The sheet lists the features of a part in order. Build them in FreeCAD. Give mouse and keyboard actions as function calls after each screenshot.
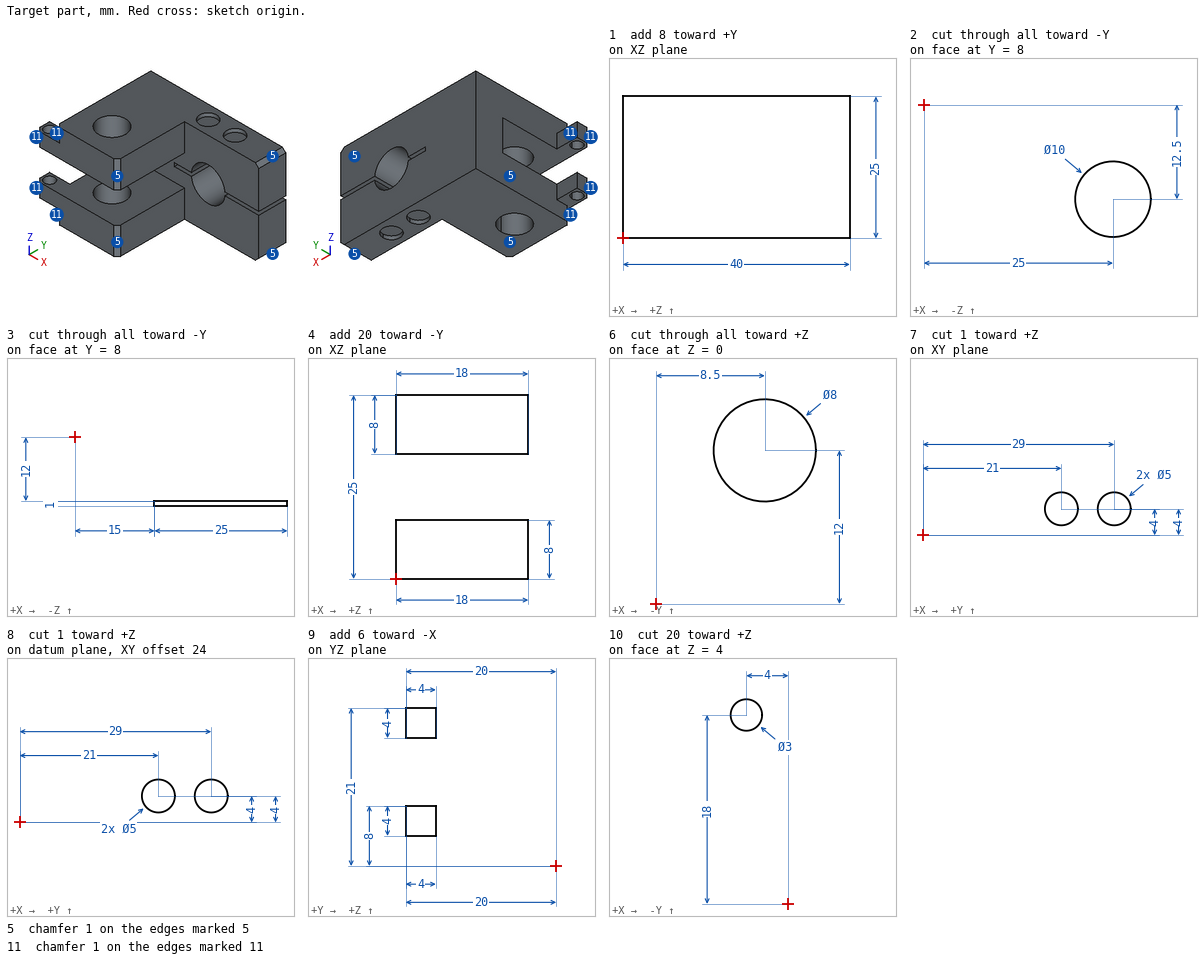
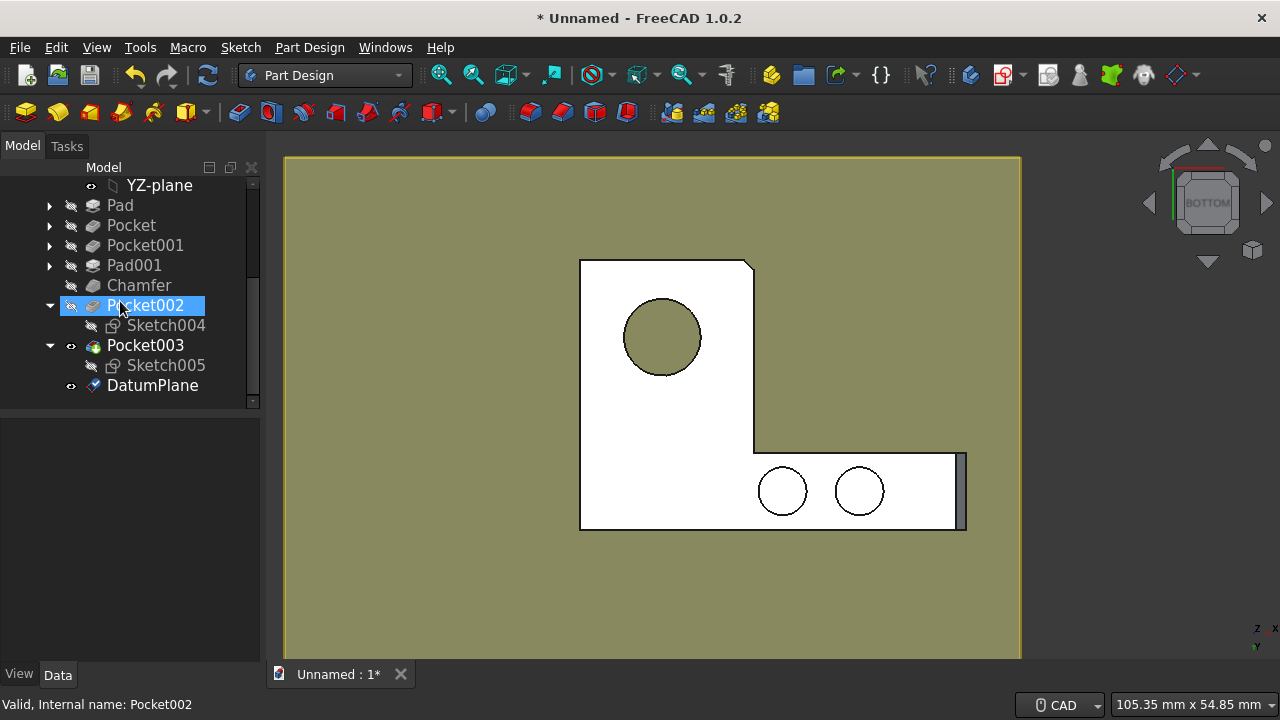
click(116, 386)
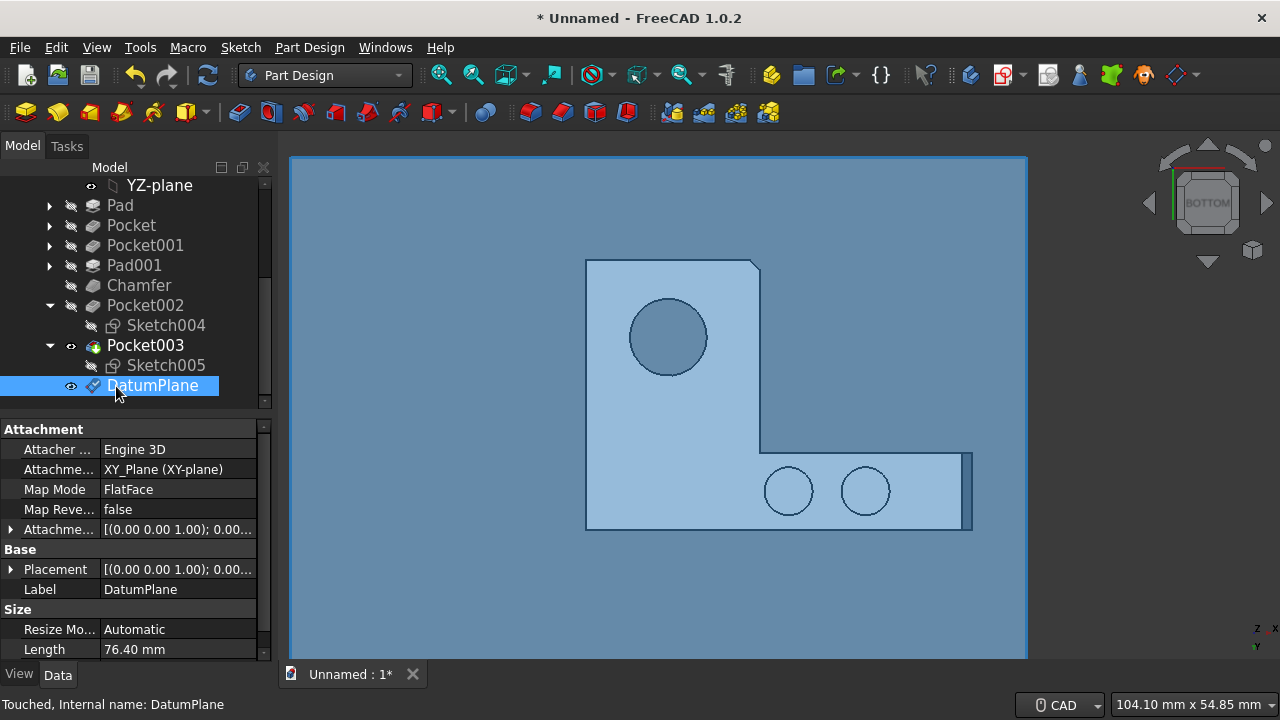
click(1004, 76)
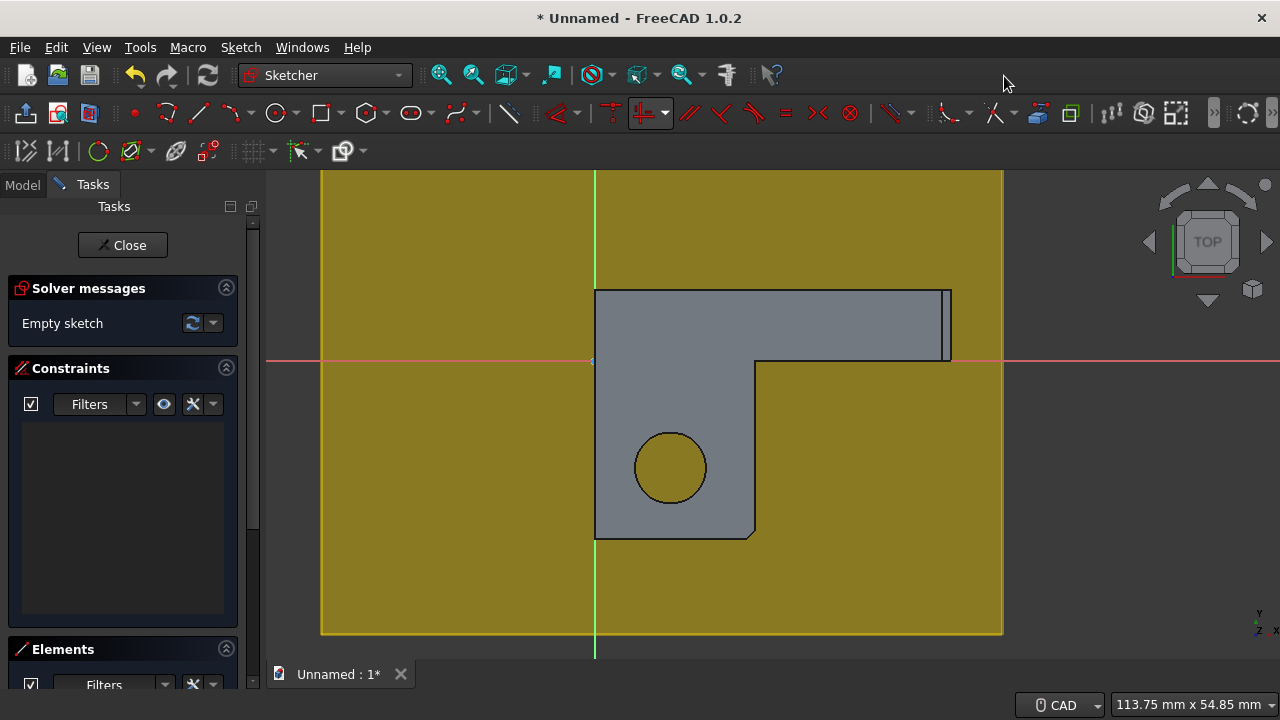
click(90, 114)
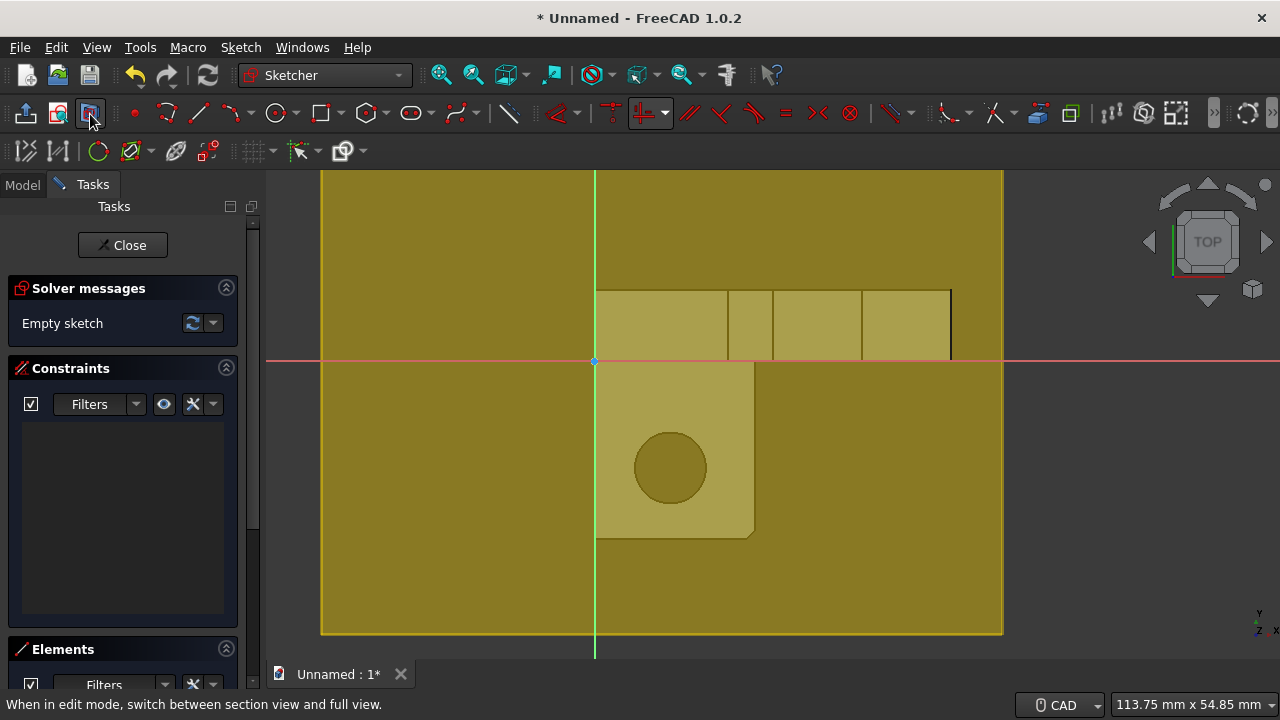
scroll(760, 265, up, 4)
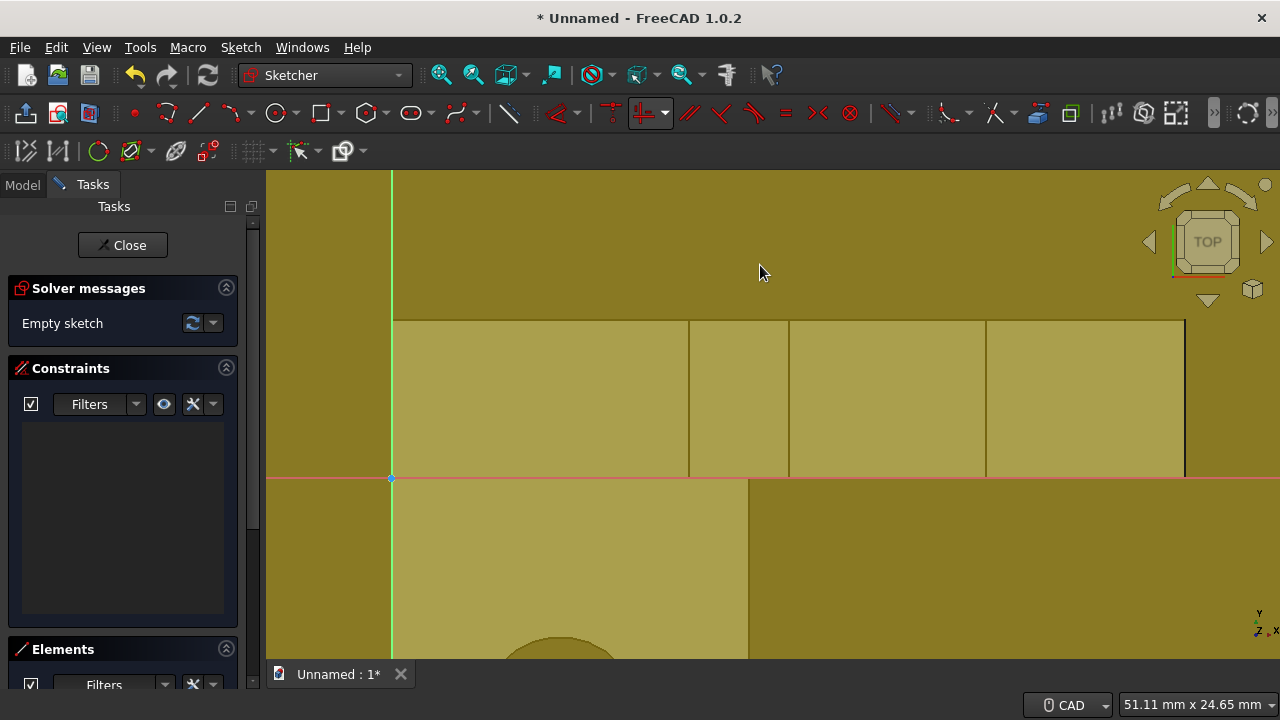
click(276, 114)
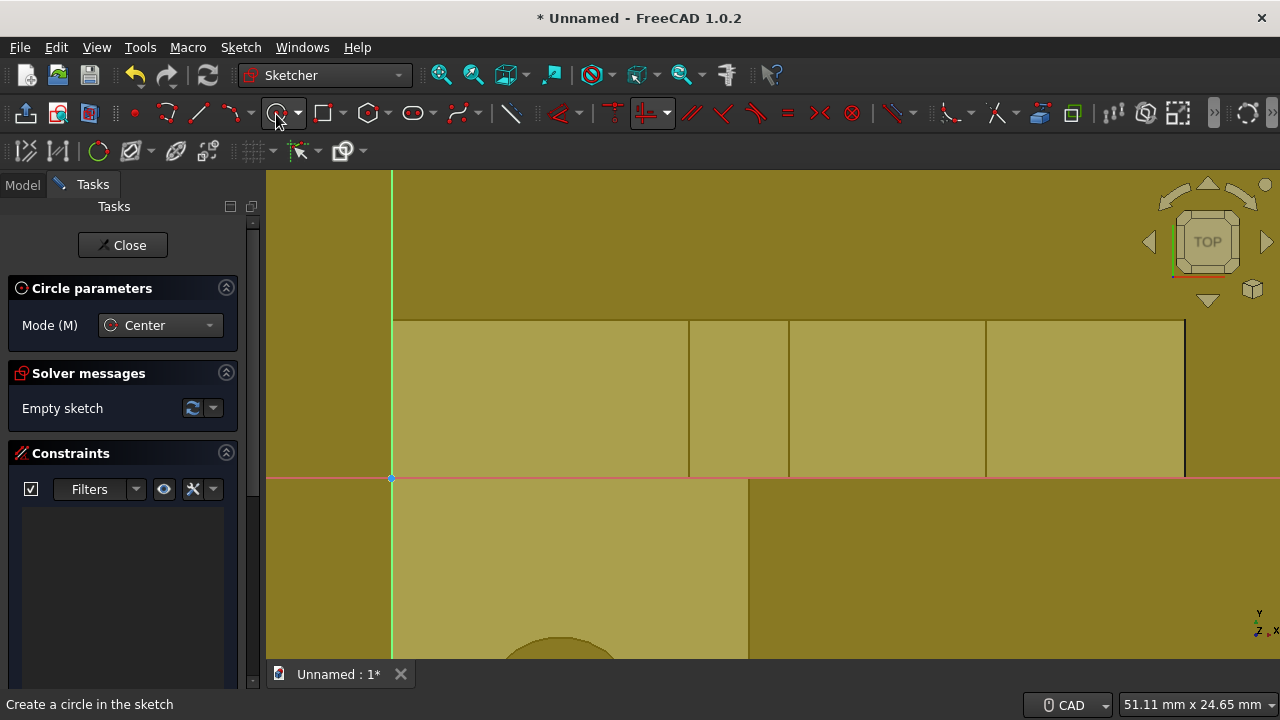
click(808, 399)
click(843, 364)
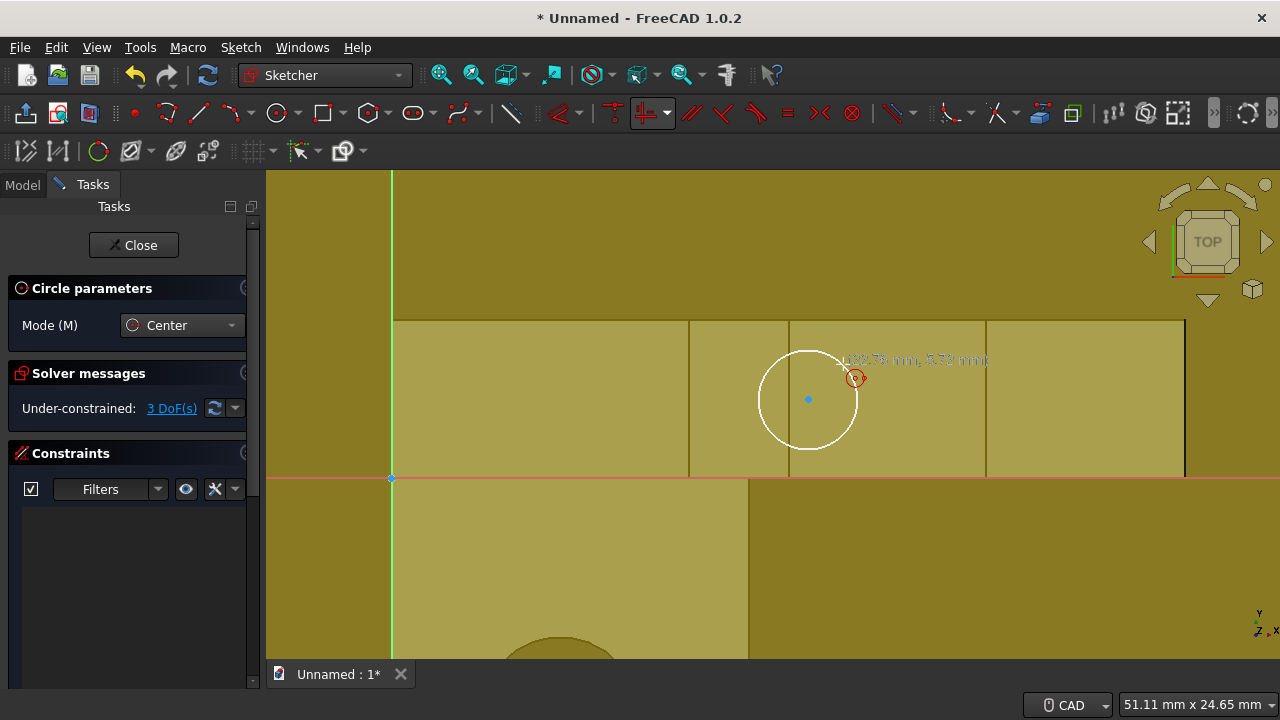
click(967, 399)
click(1002, 364)
key(Escape)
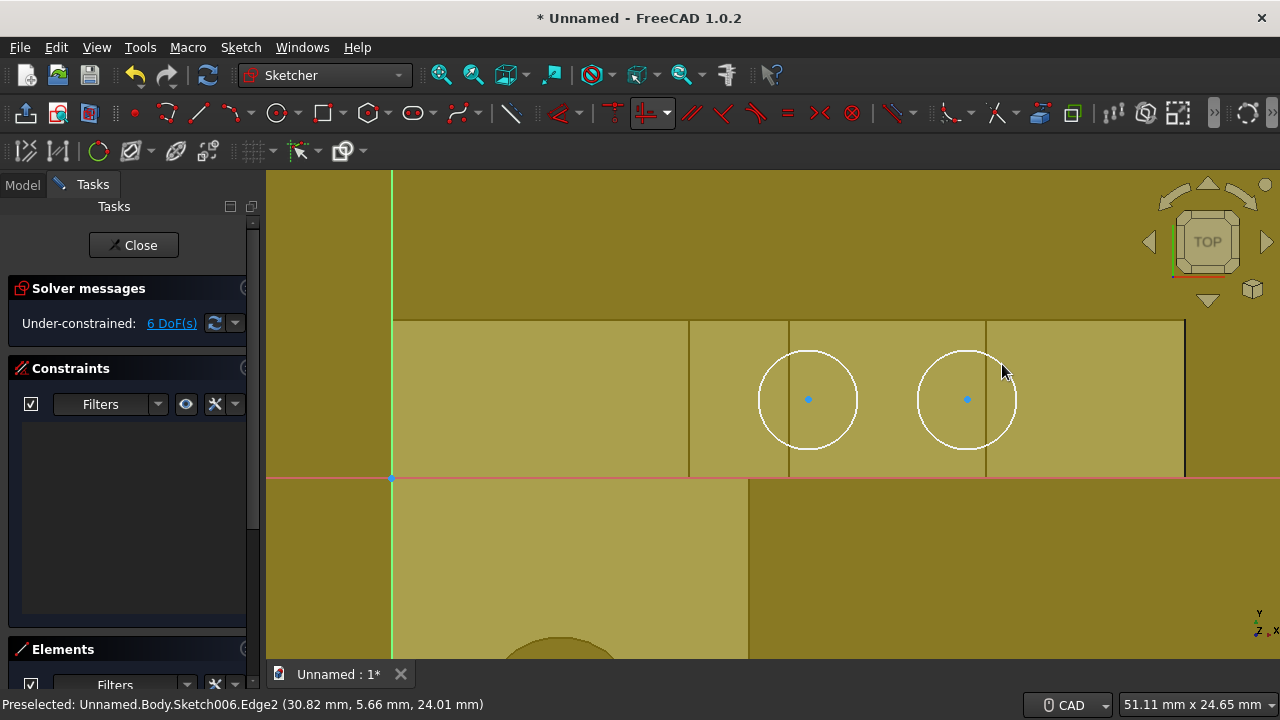
click(843, 365)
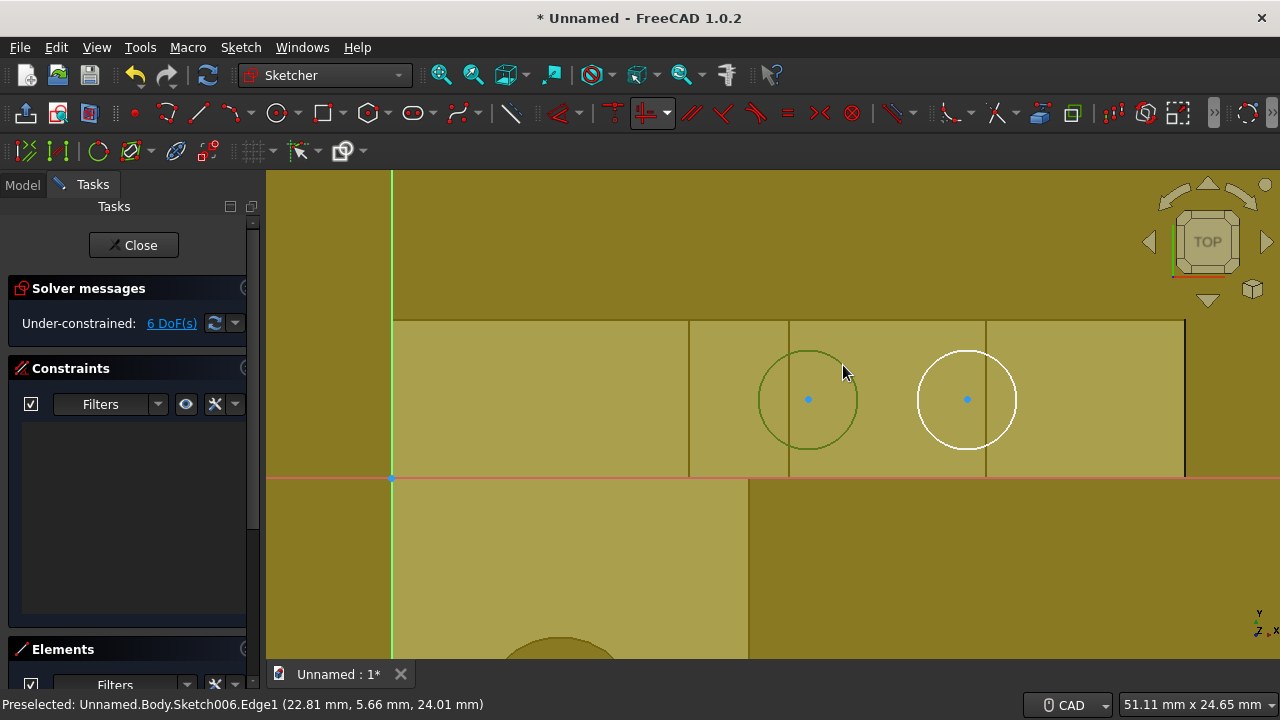
click(1002, 365)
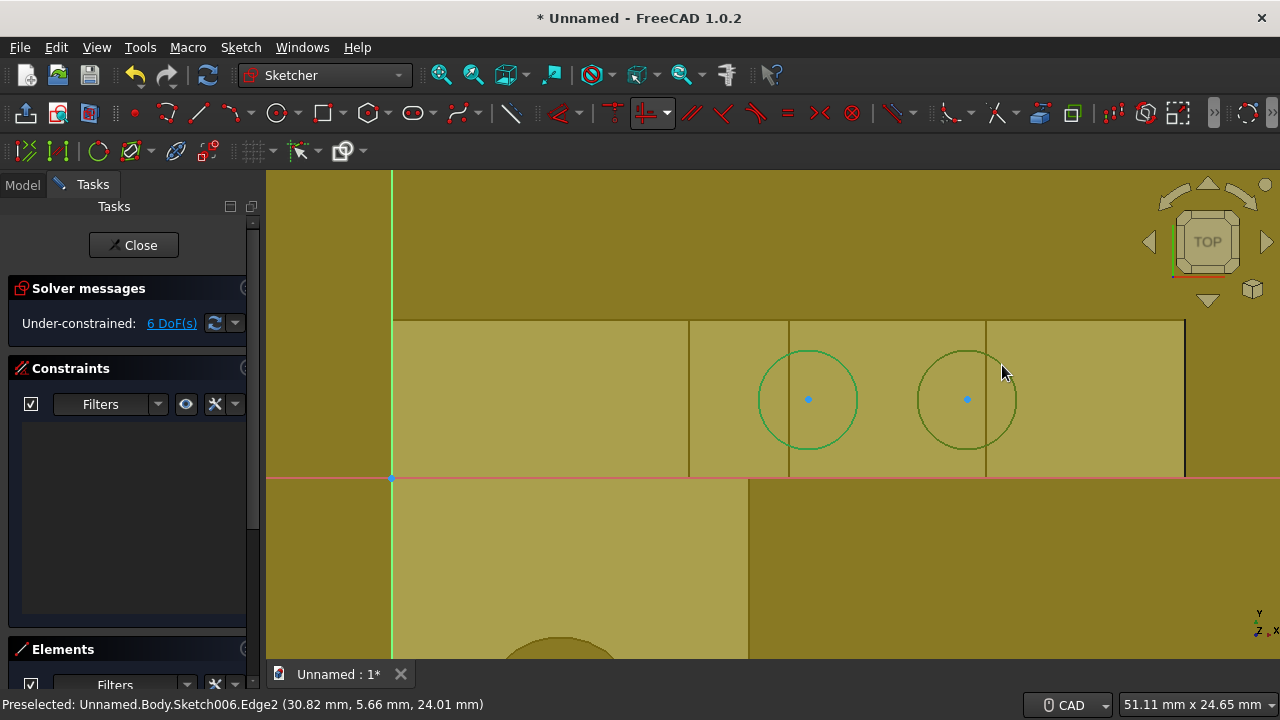
click(788, 114)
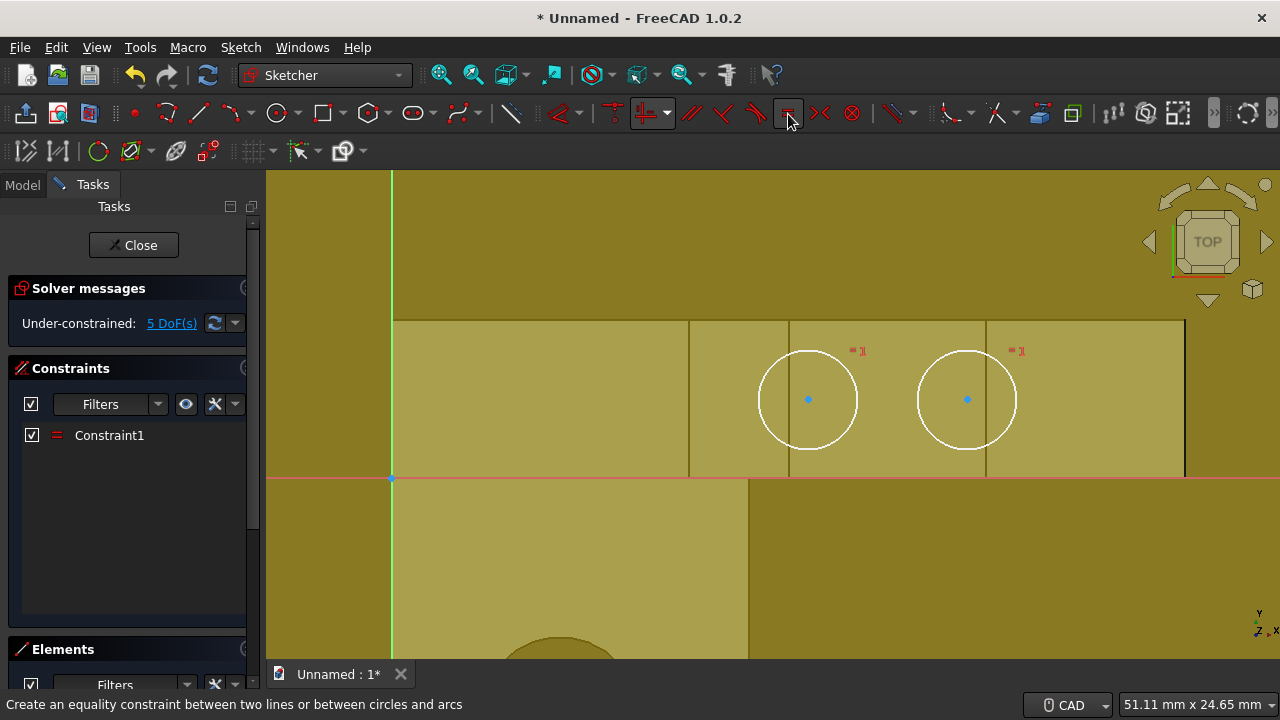
click(558, 114)